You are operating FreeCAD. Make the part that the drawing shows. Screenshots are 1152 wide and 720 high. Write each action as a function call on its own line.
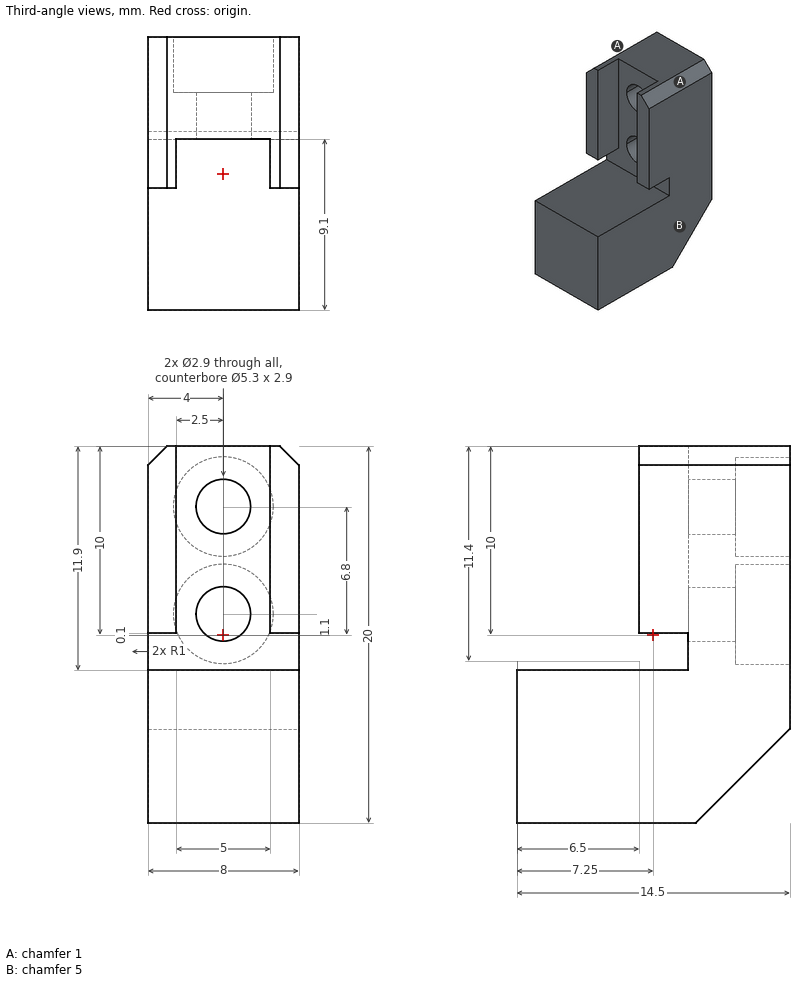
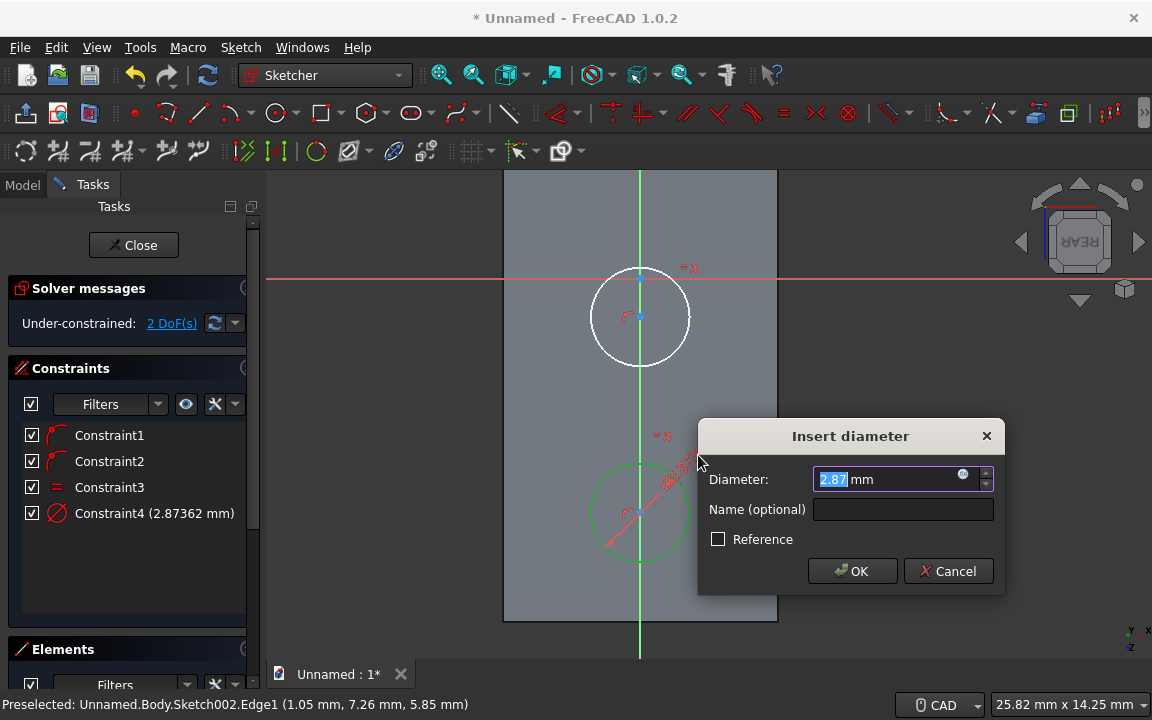
text(2.9)
key(Return)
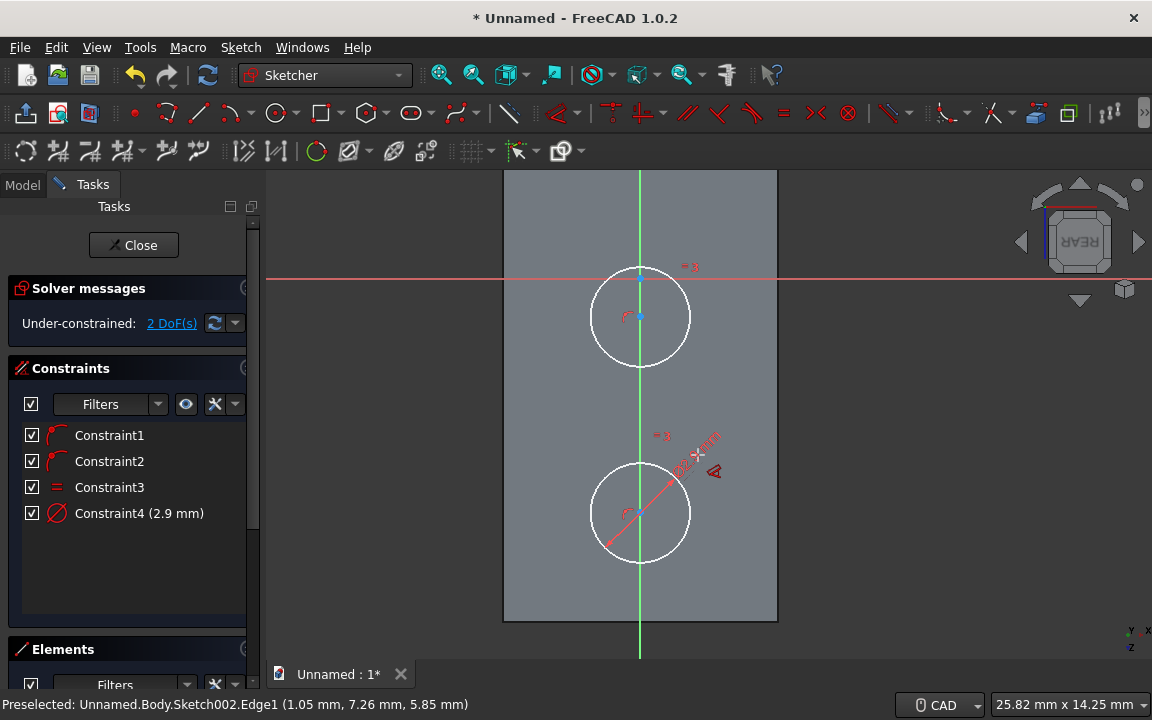
click(640, 513)
click(674, 396)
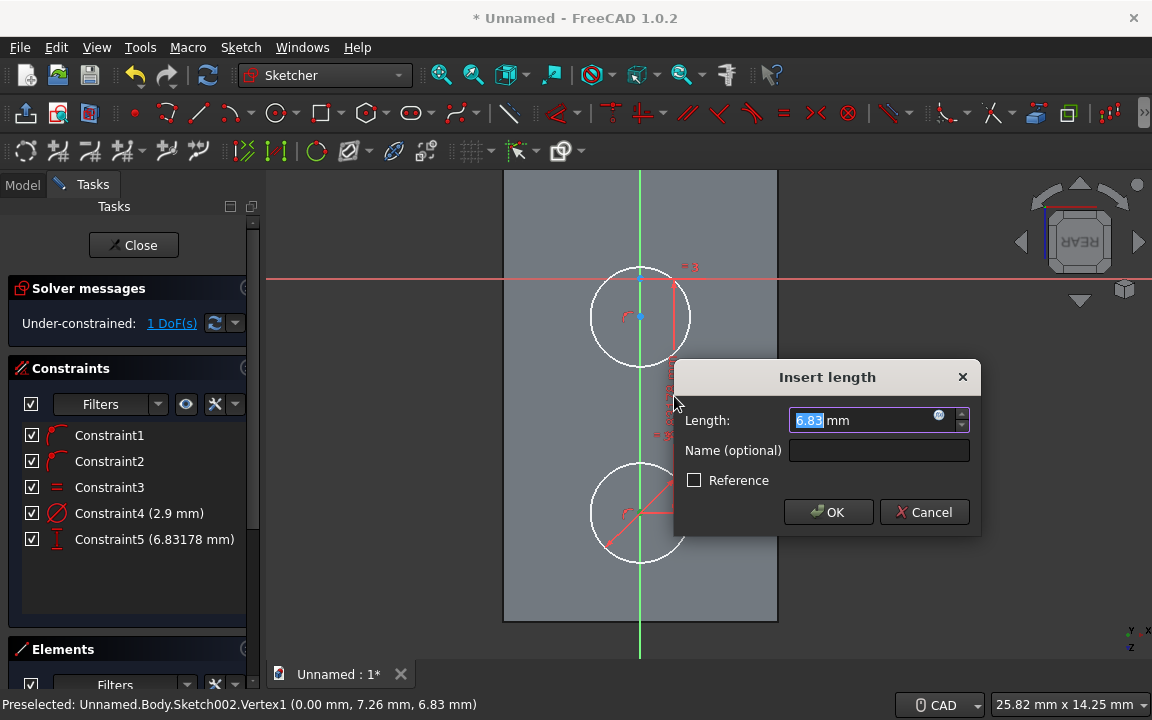
text(6.8)
key(Return)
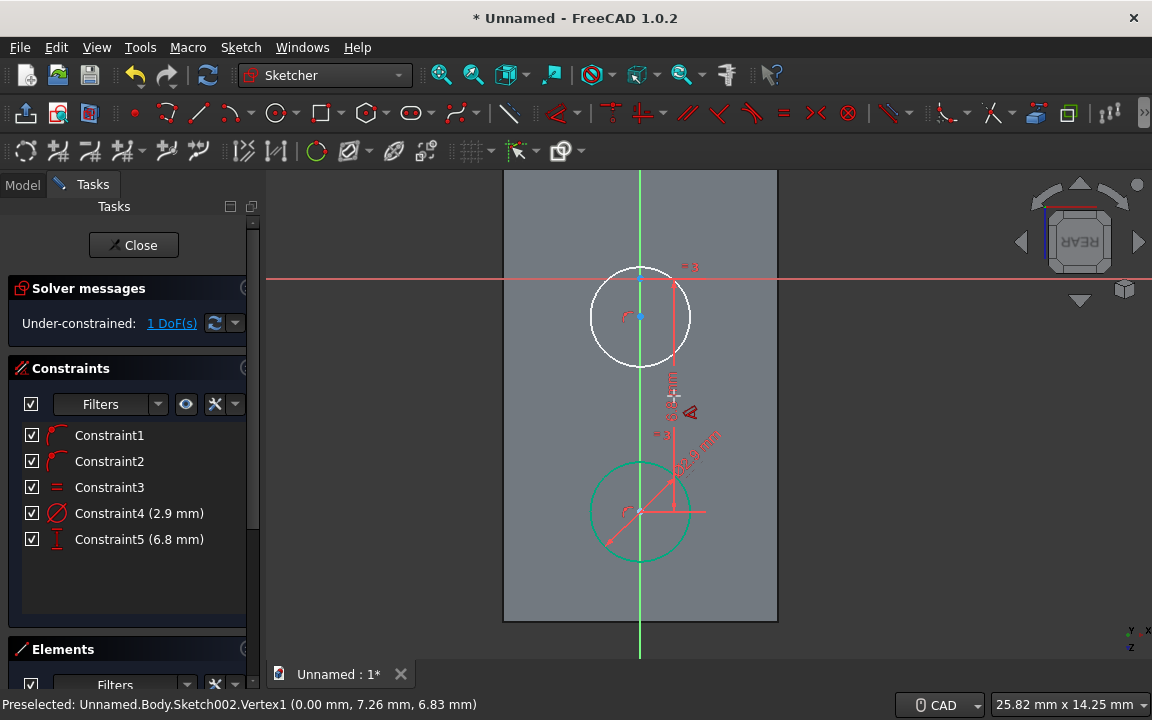
click(640, 317)
click(674, 307)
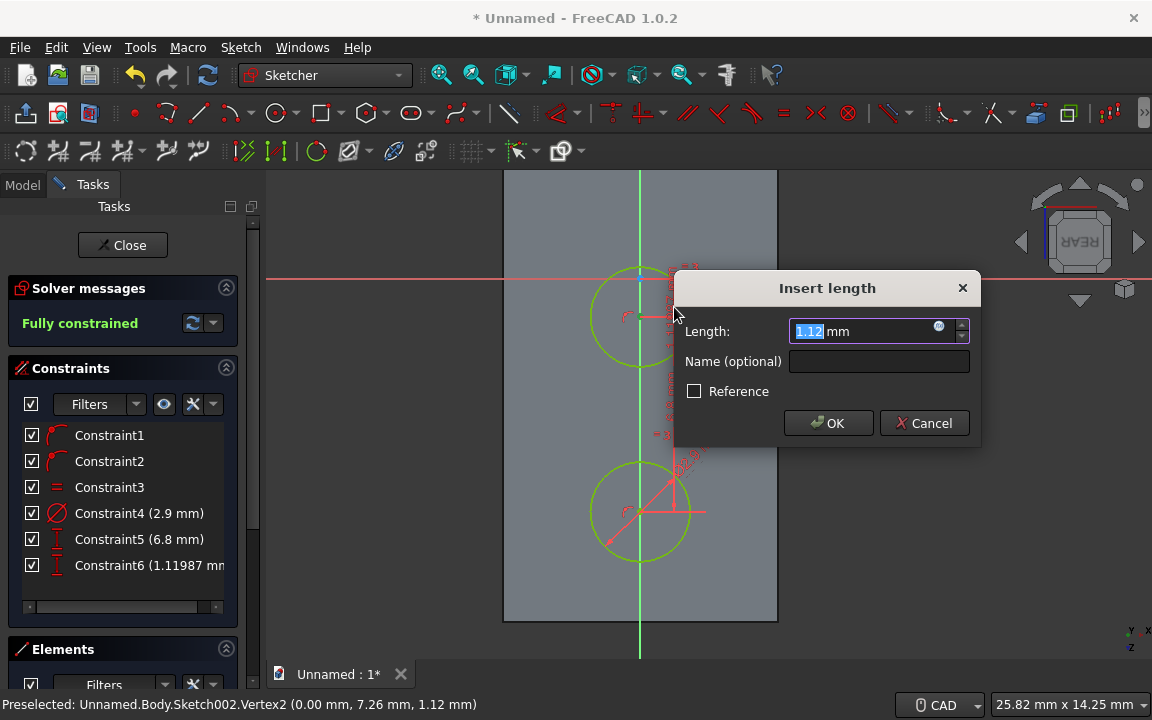
text(1.1)
key(Return)
key(Escape)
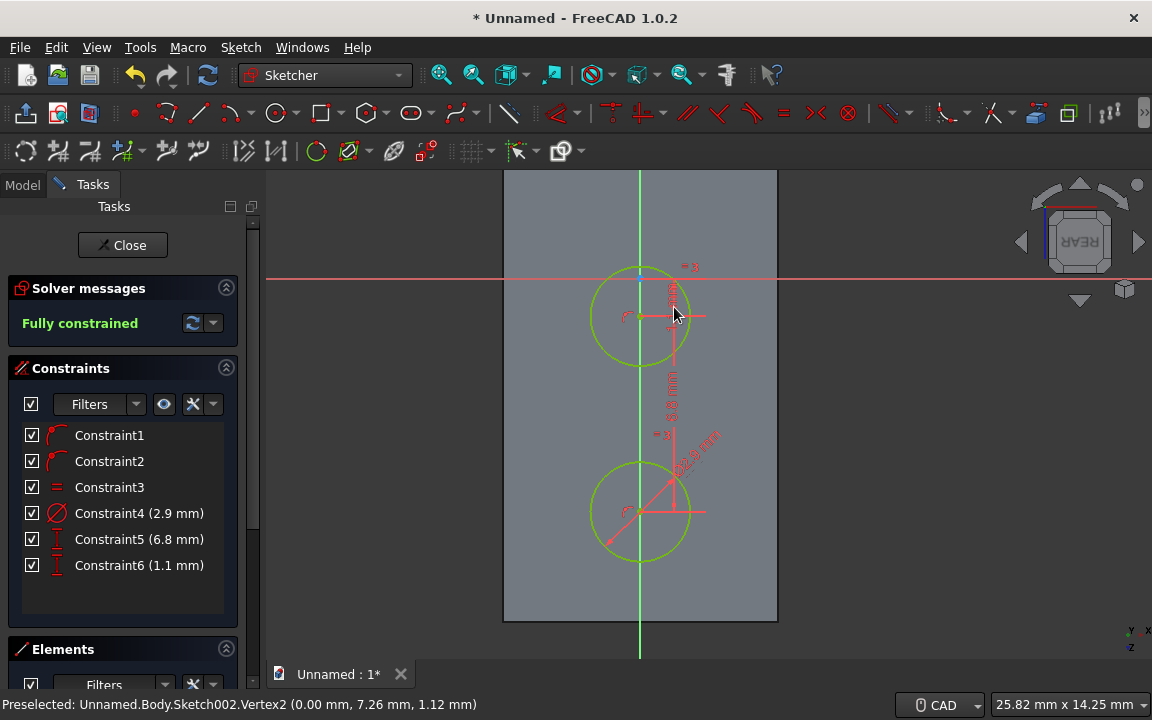
click(123, 245)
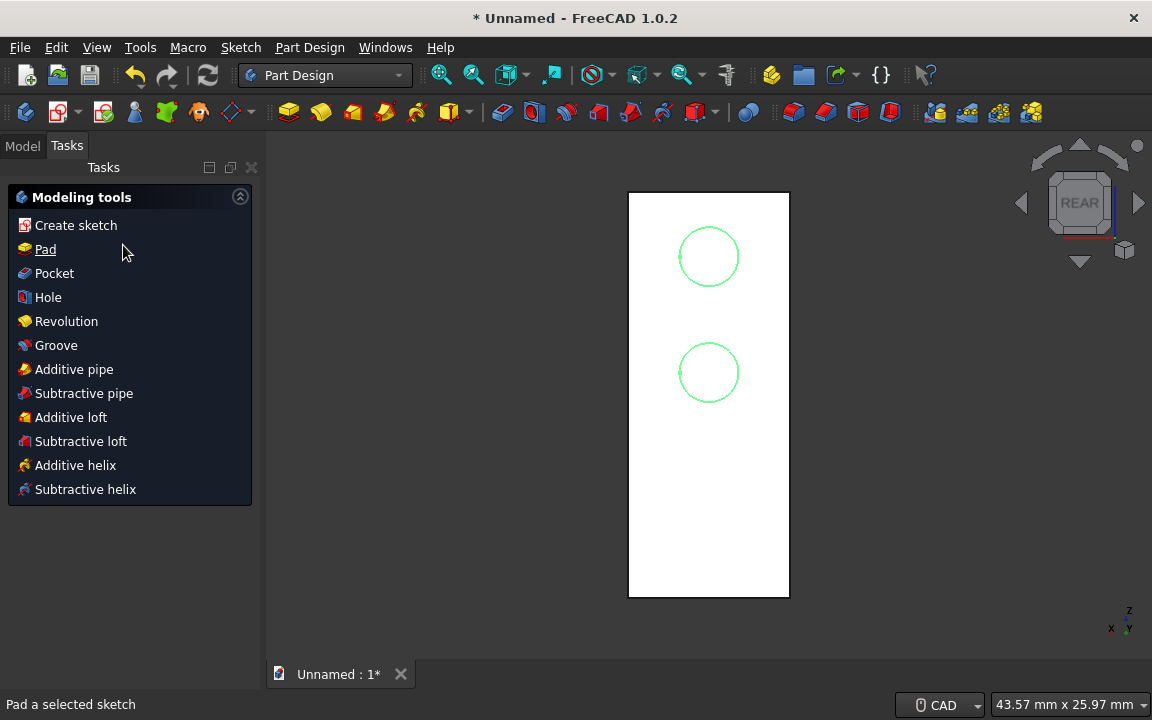
click(536, 112)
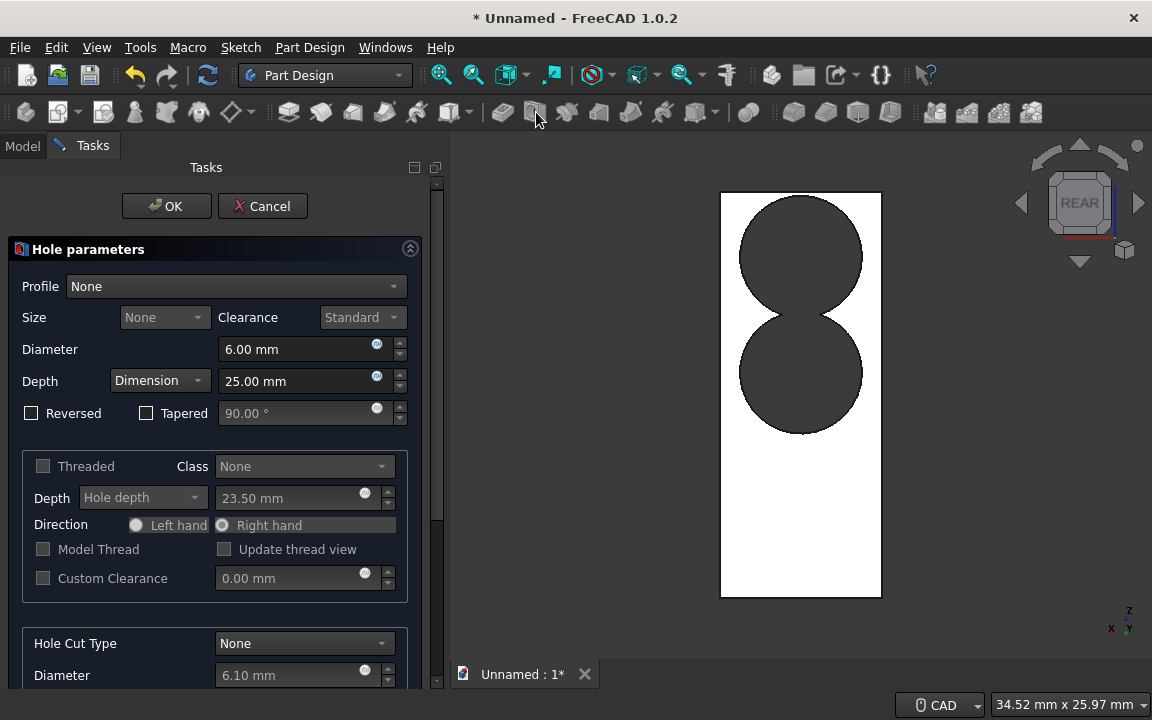
triple_click(305, 349)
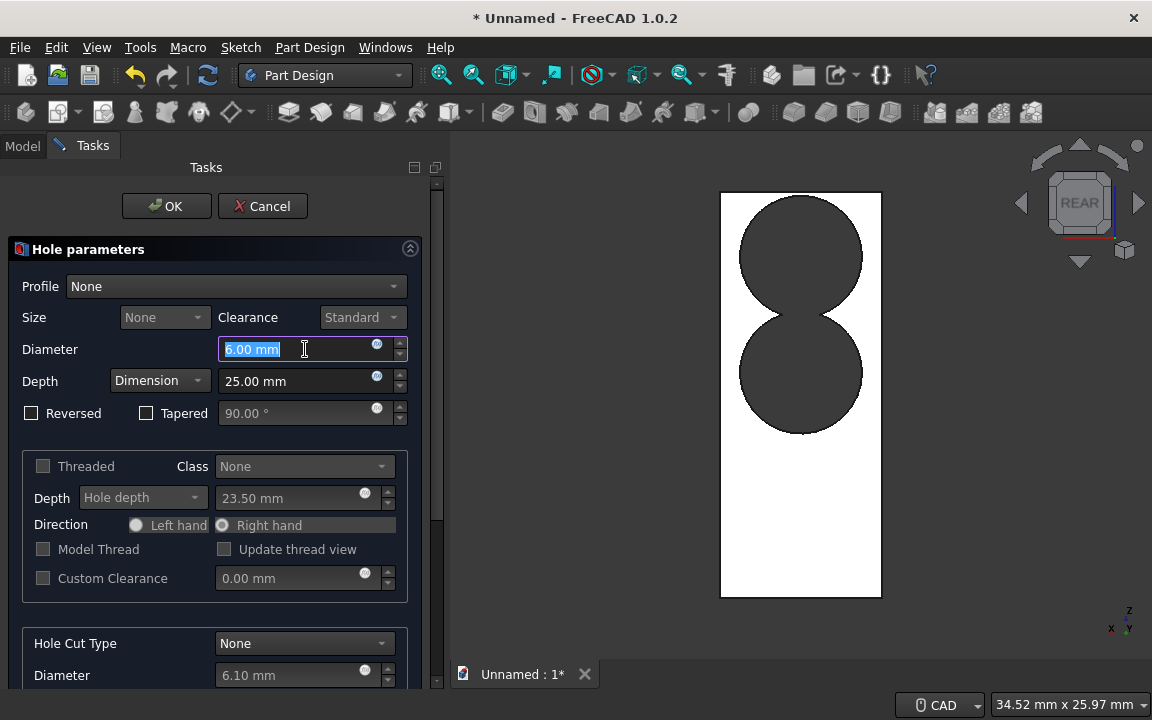
text(2.9)
key(Tab)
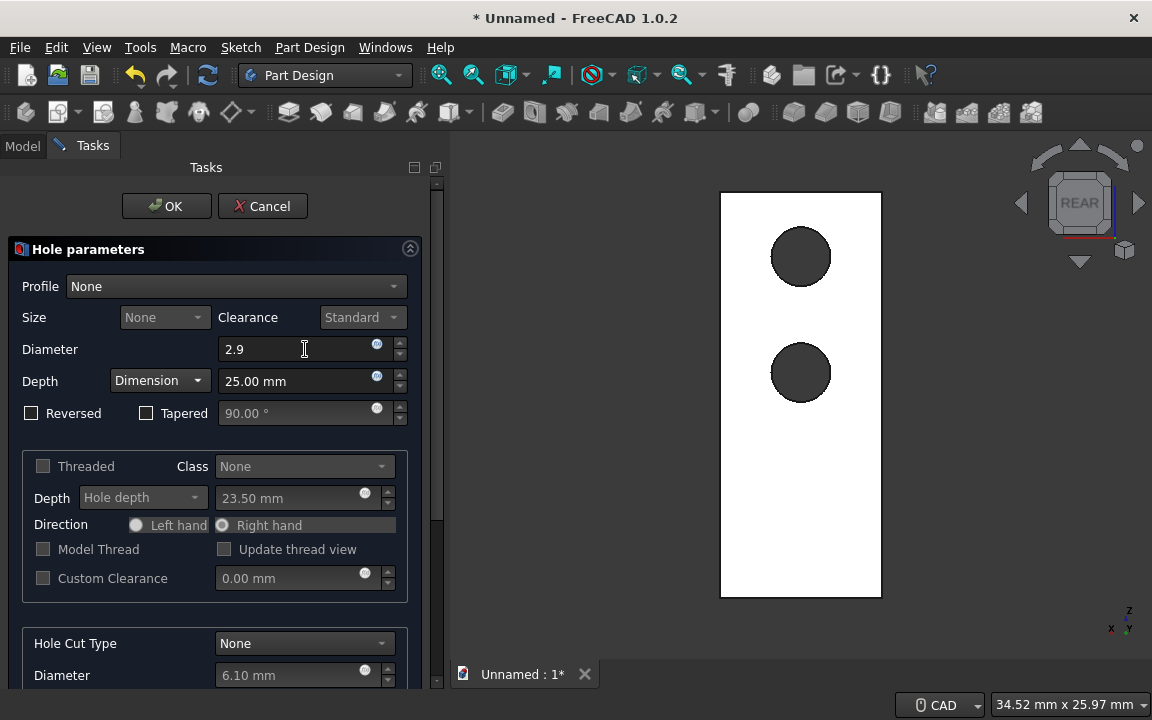
click(161, 380)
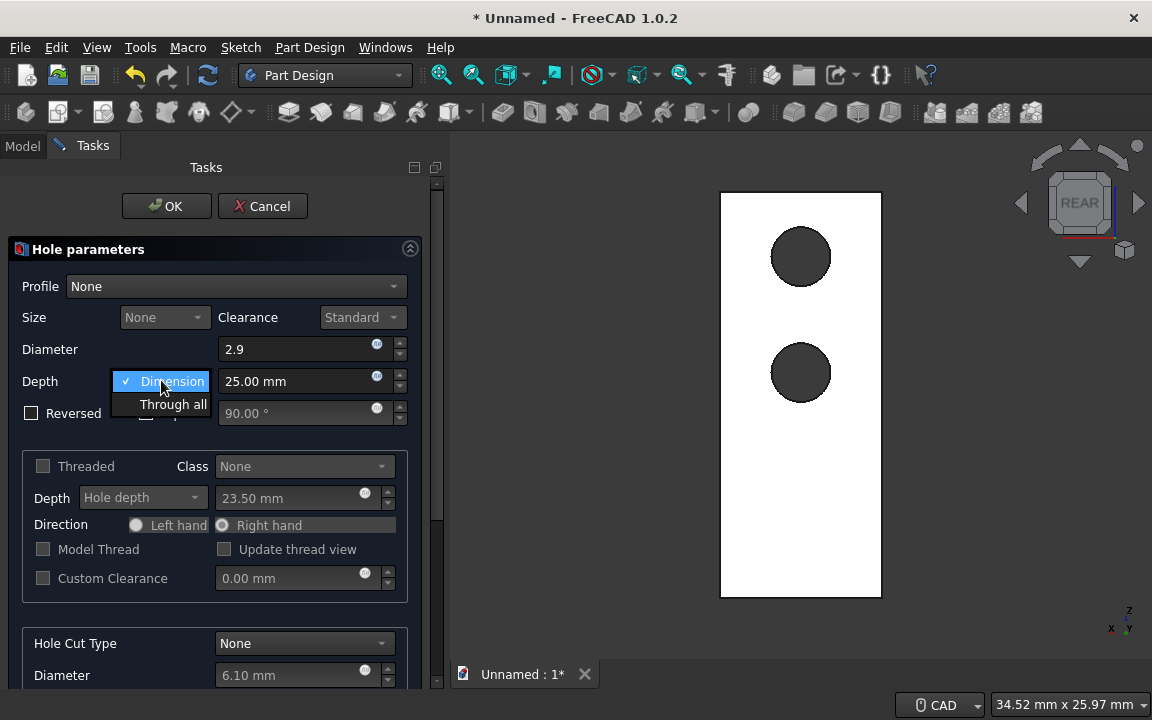
click(160, 404)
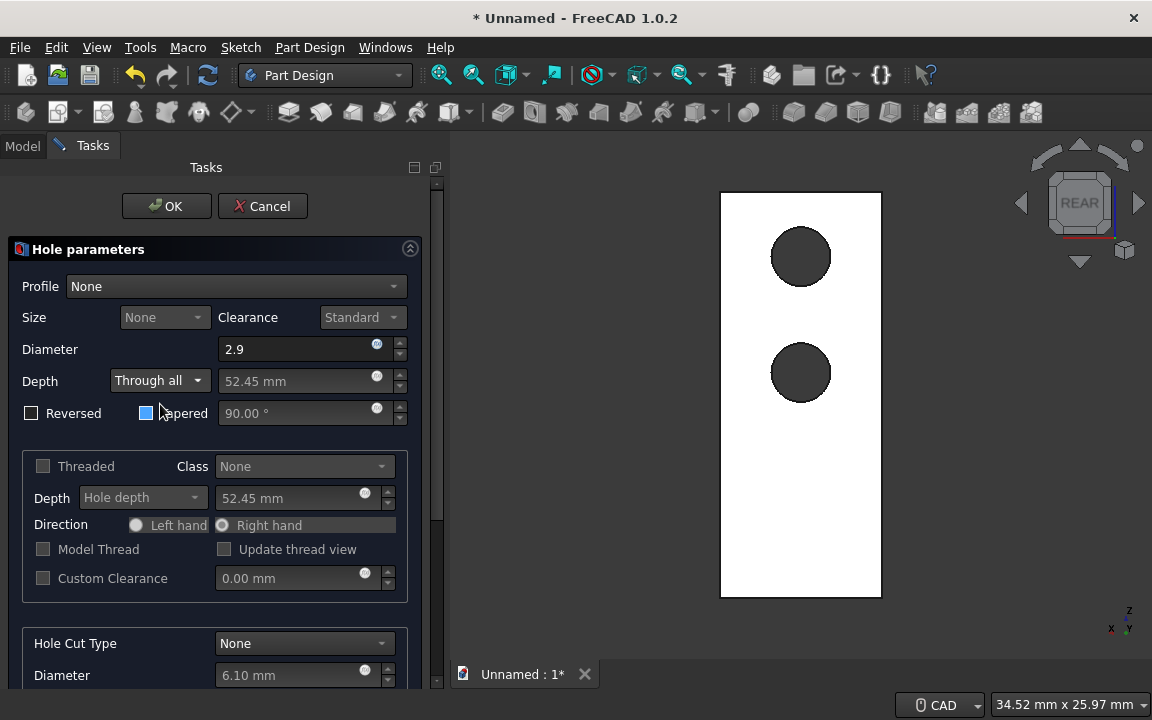
click(306, 644)